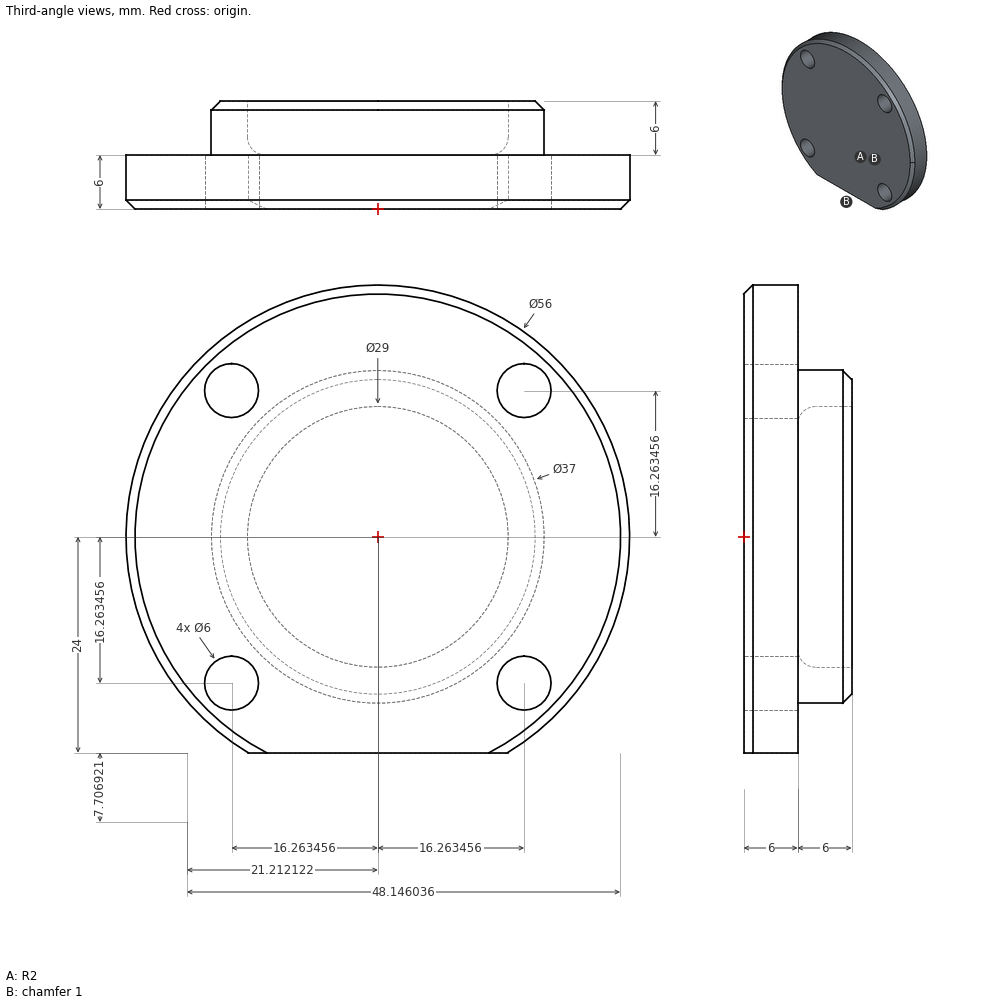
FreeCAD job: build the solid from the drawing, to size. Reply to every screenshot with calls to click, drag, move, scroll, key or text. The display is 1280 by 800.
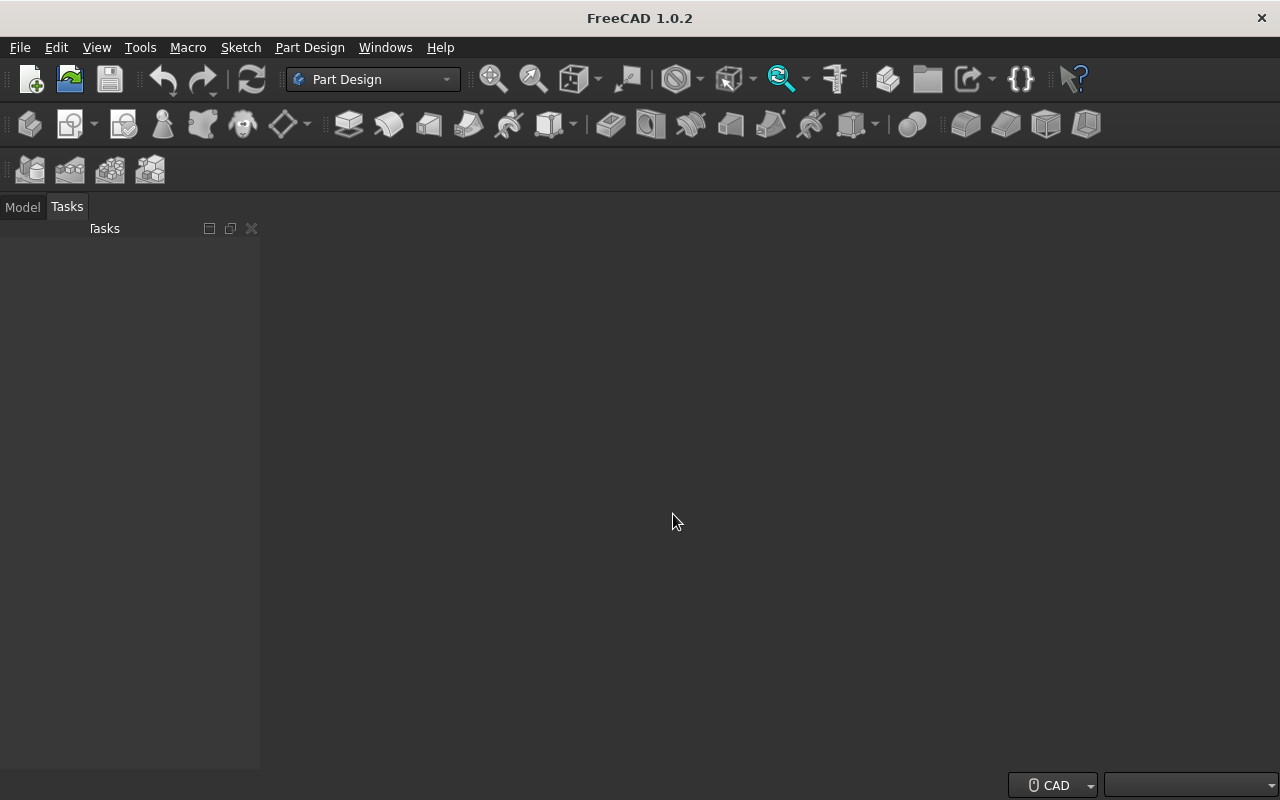
key(ctrl+n)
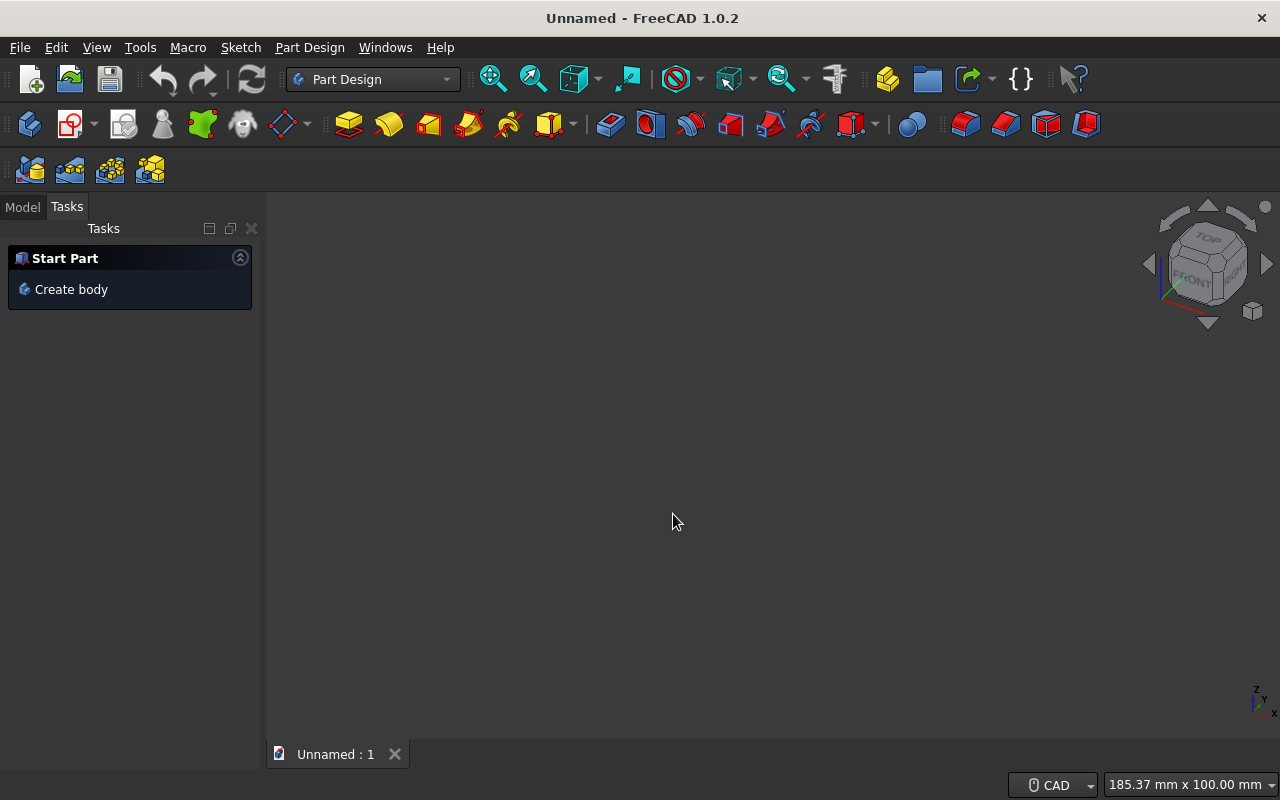
click(70, 124)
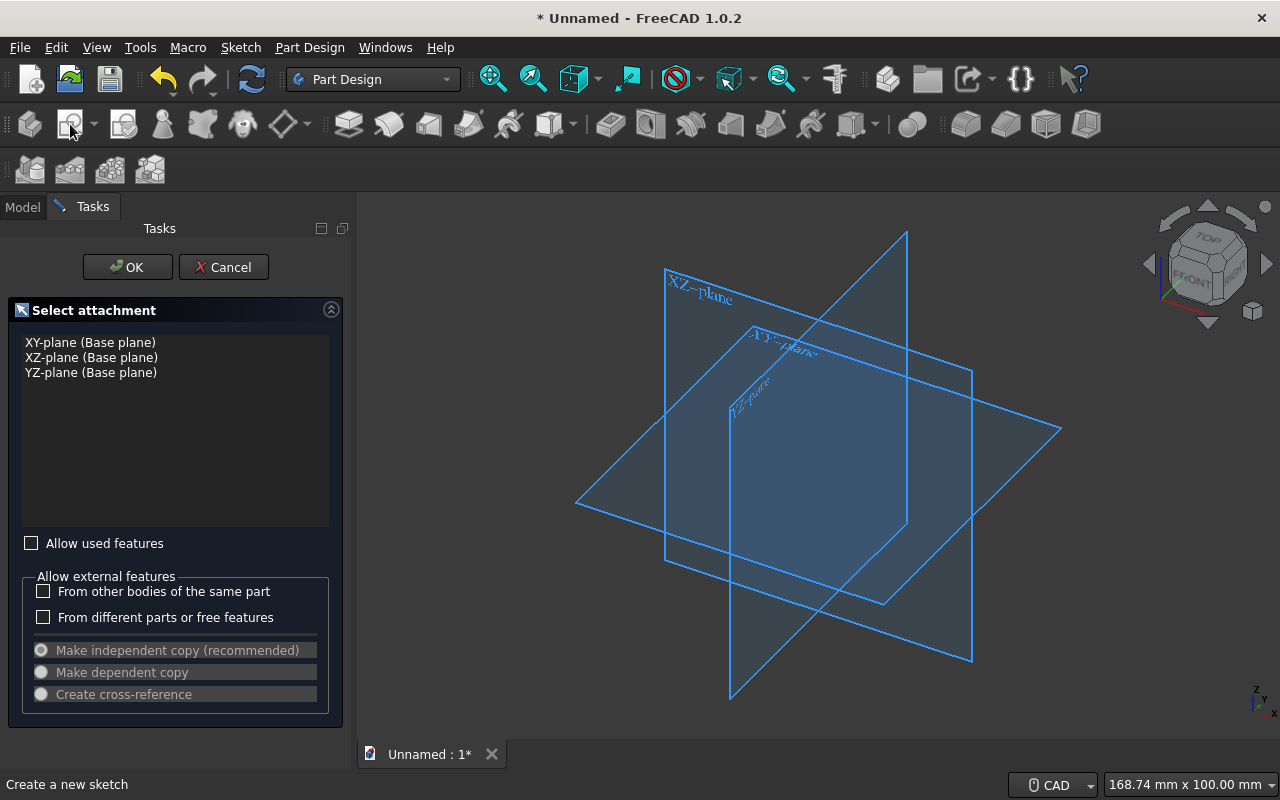
click(82, 358)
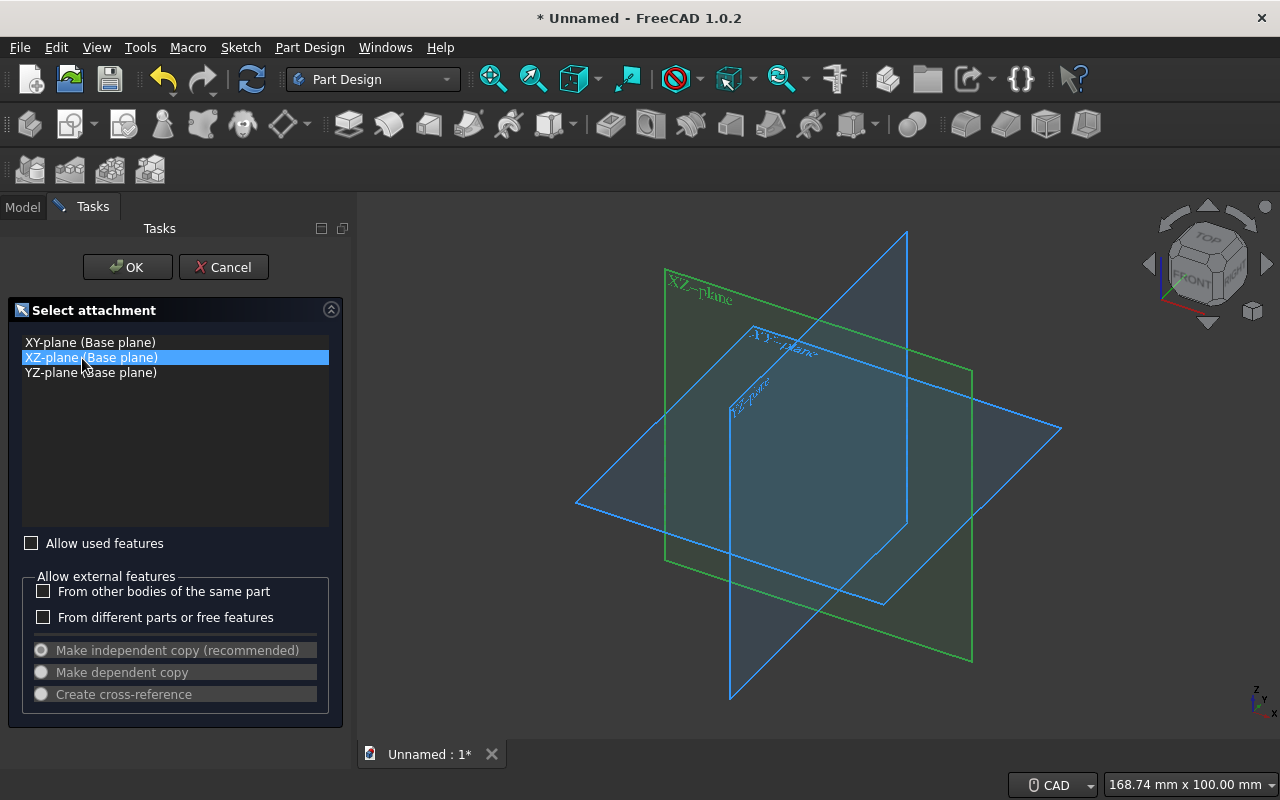
click(128, 267)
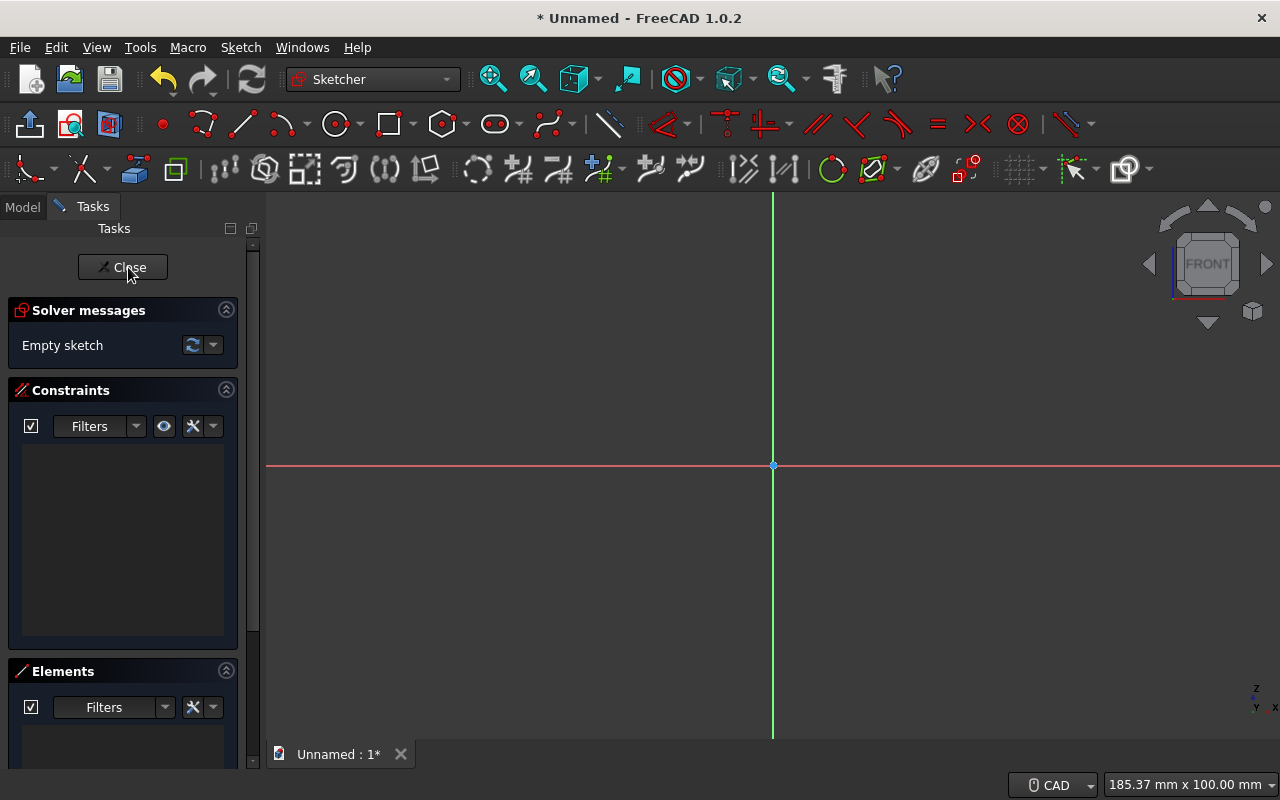
key(g)
key(c)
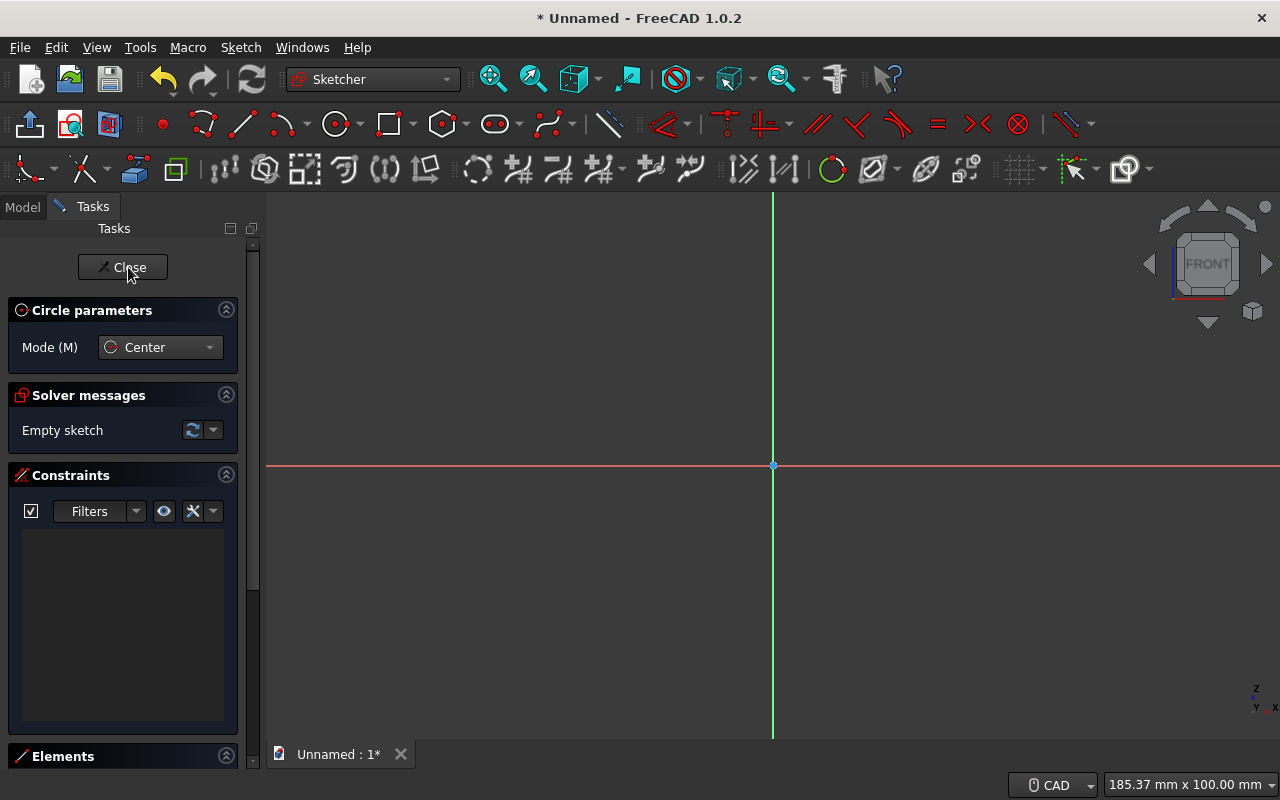
click(773, 466)
click(881, 357)
key(Escape)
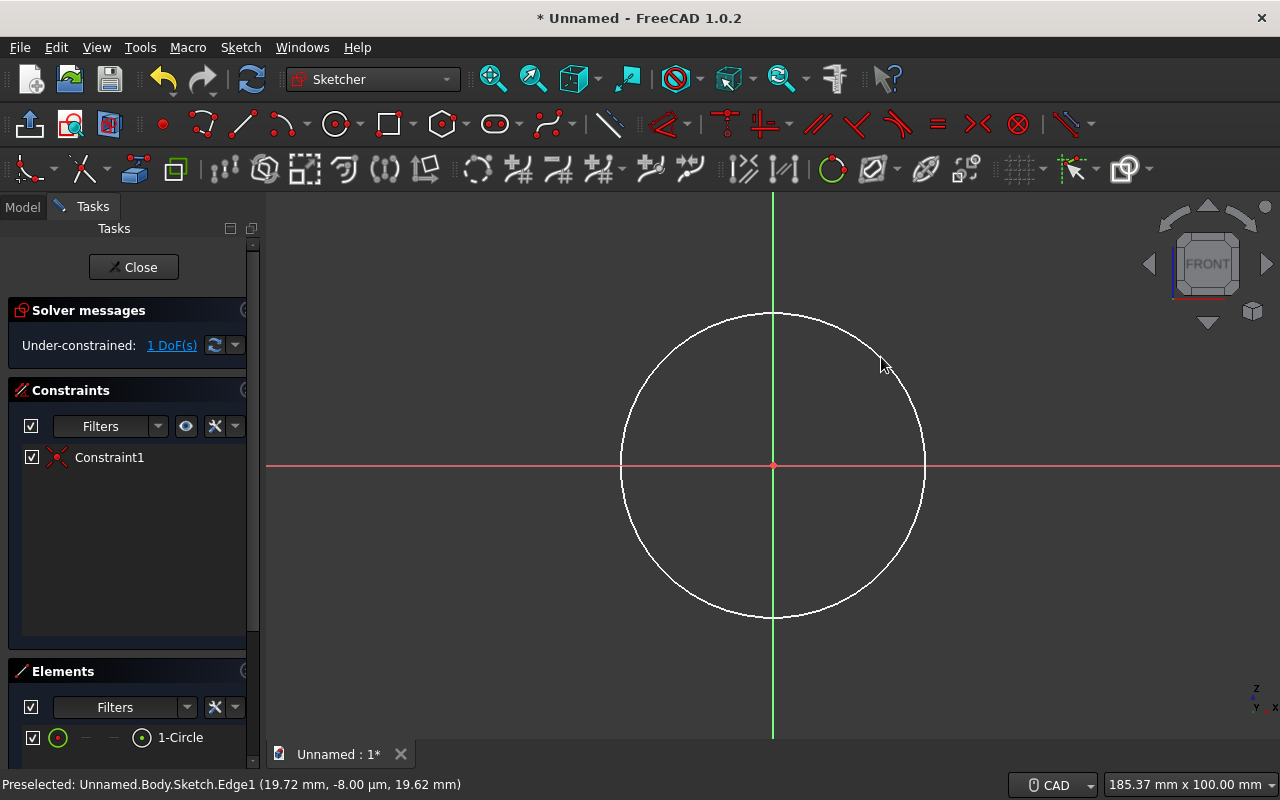
key(d)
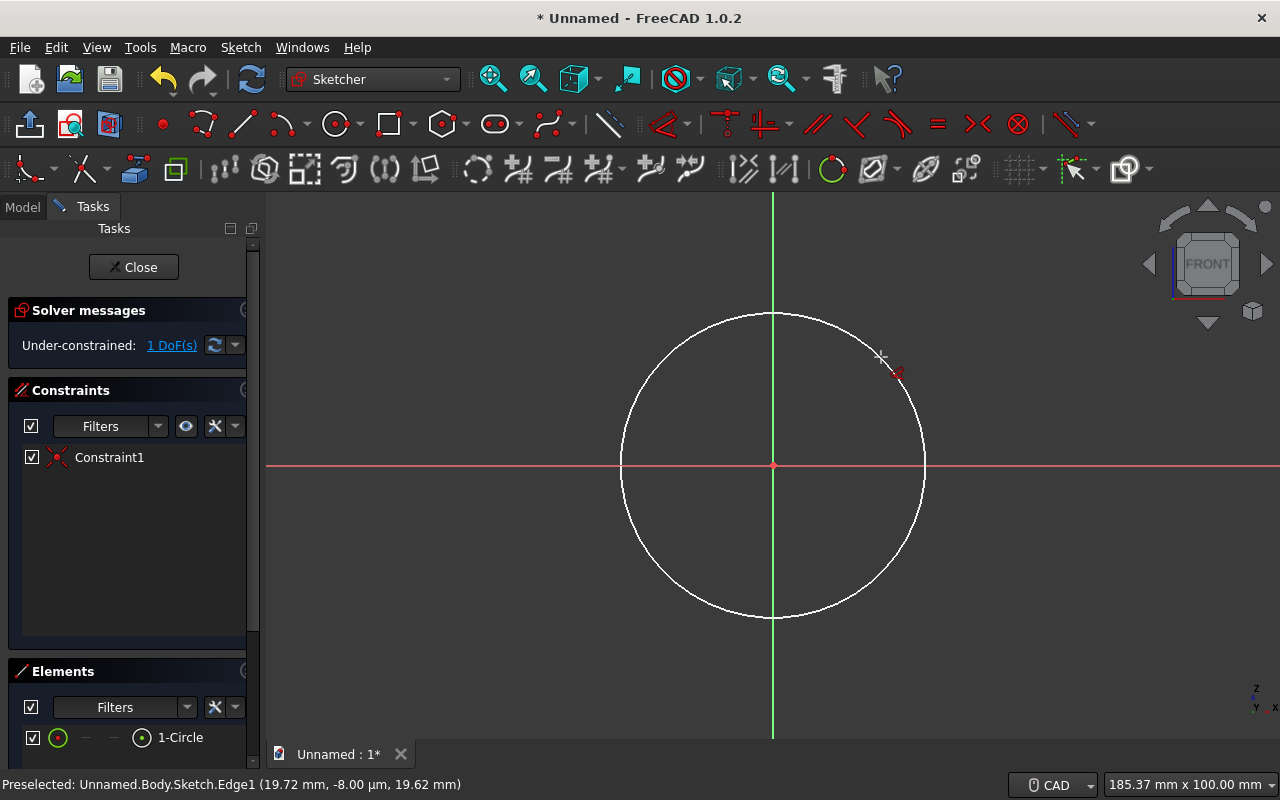
click(880, 357)
click(902, 334)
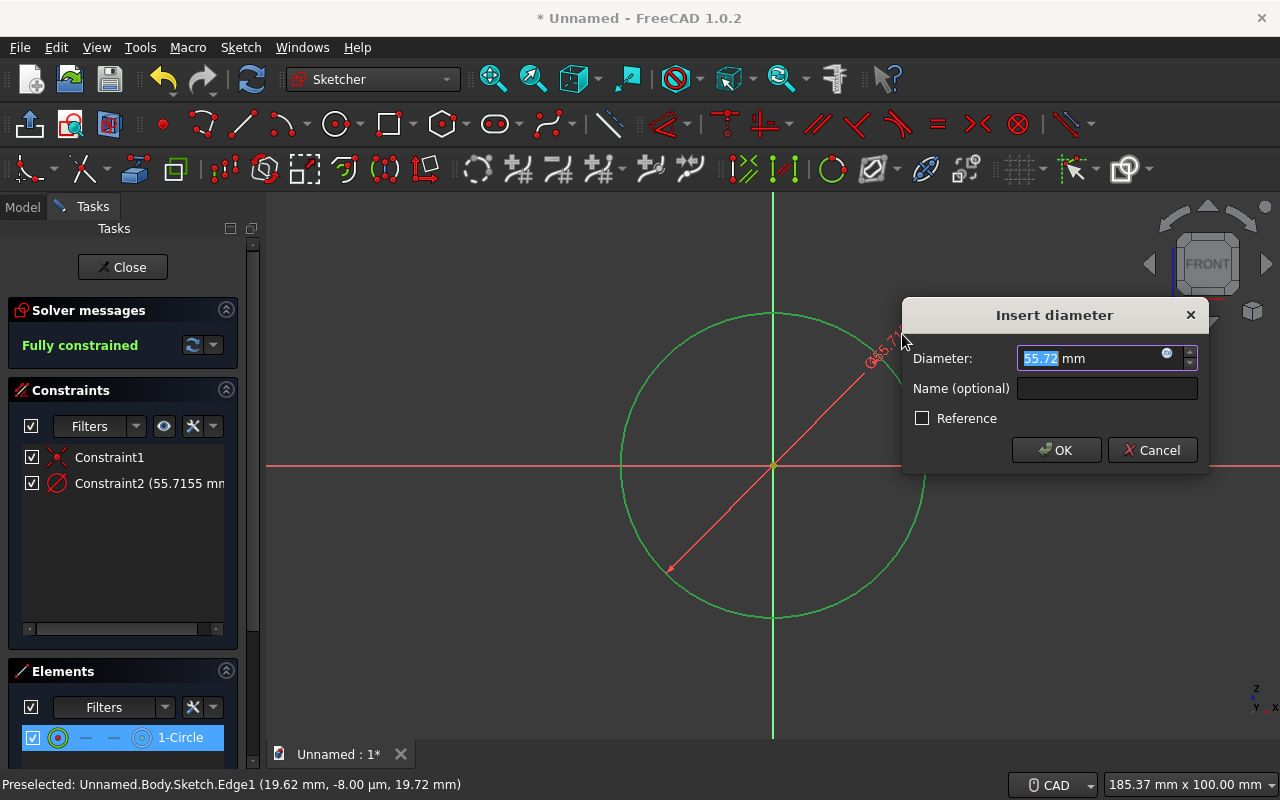
text(56)
key(Return)
key(Escape)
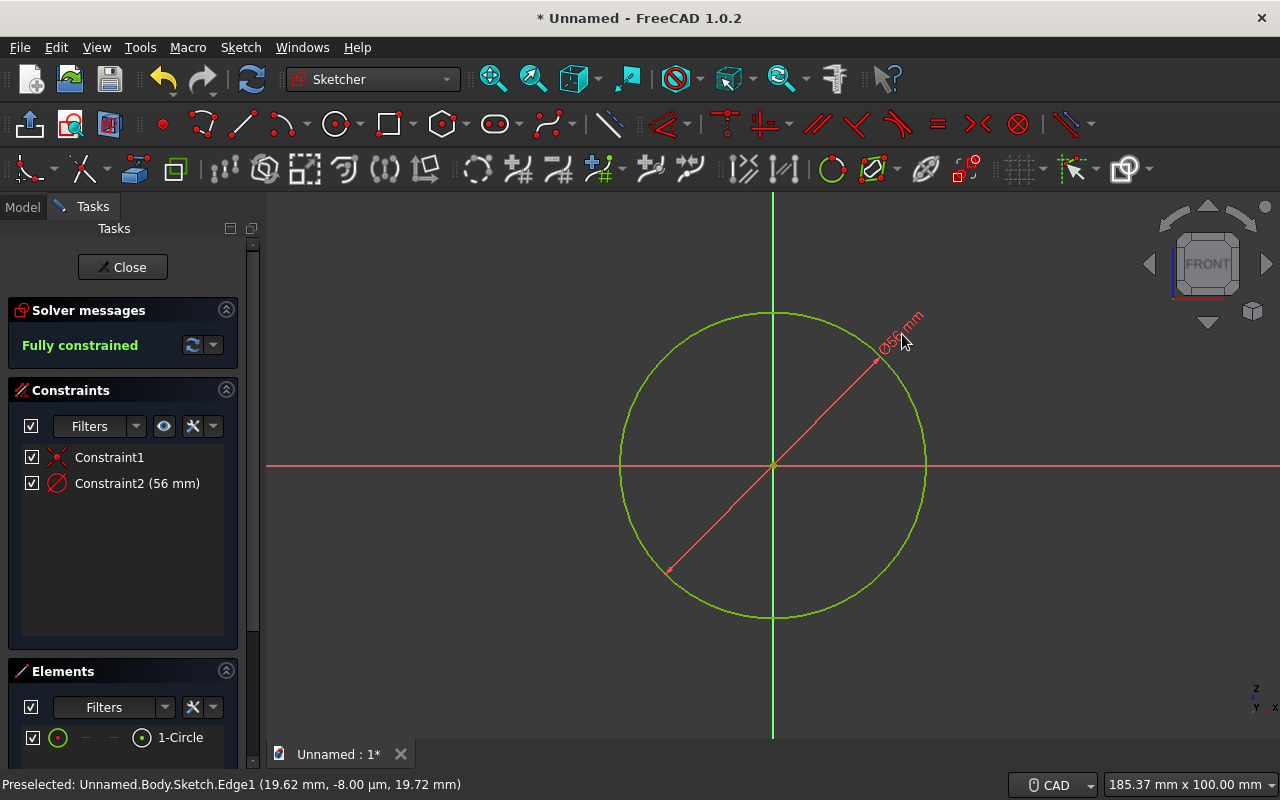
click(123, 267)